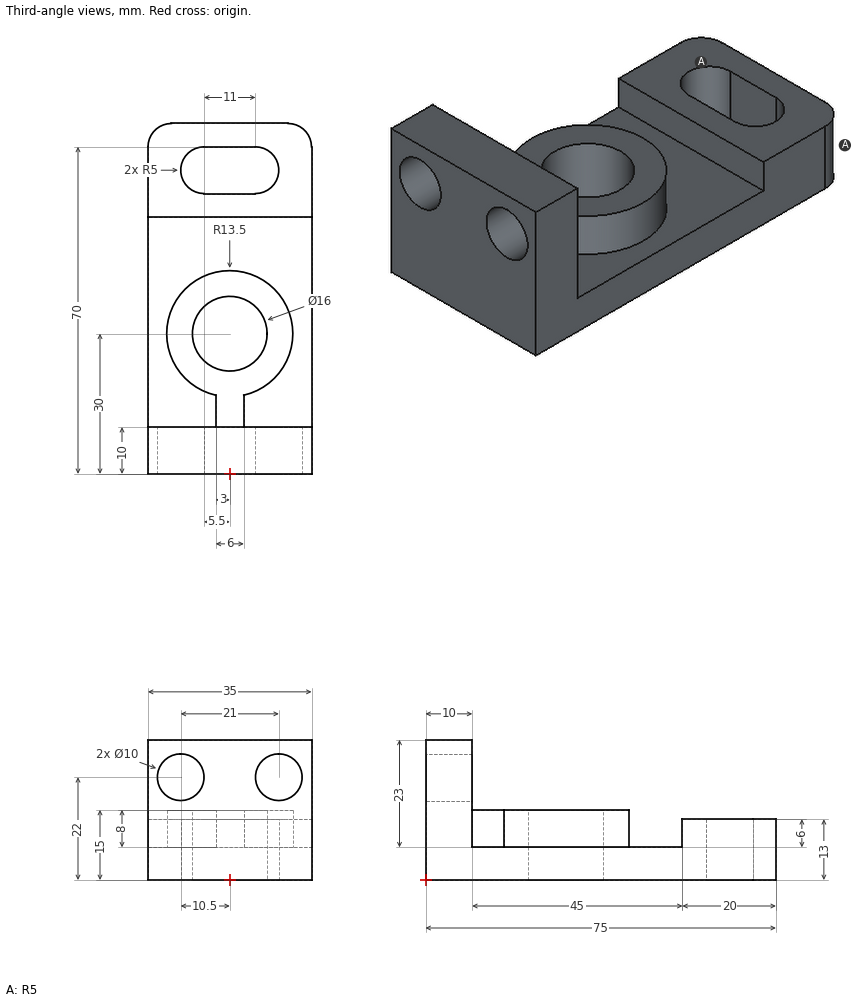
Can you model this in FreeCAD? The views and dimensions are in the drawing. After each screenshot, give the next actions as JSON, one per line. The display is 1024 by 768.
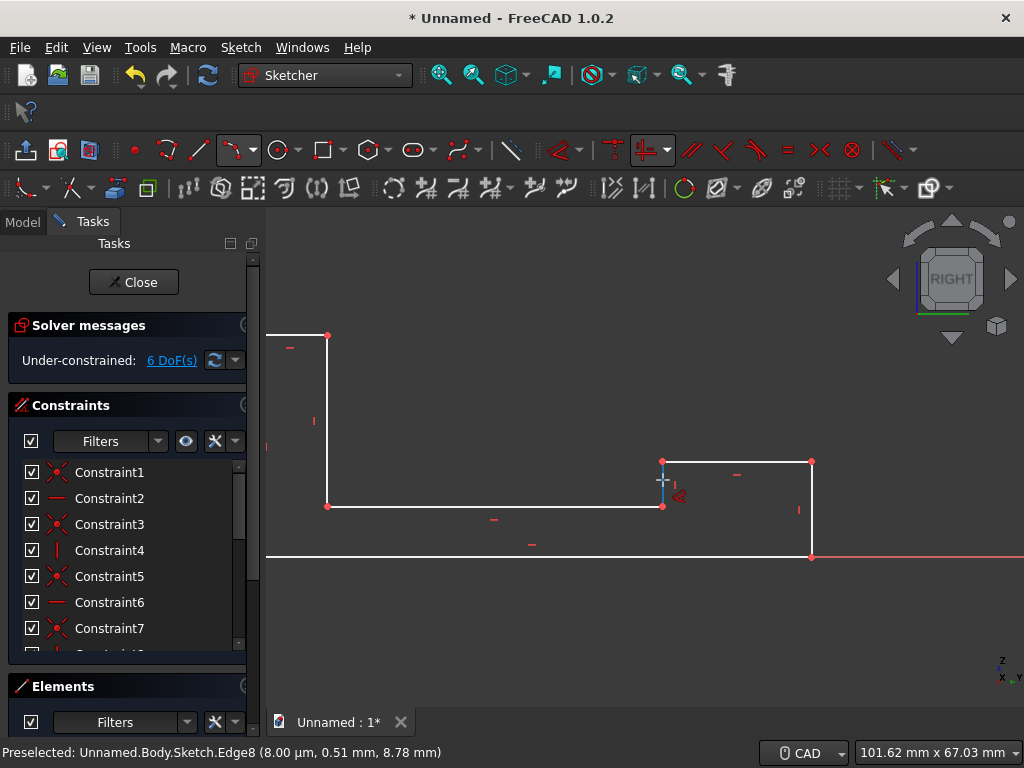
{"action": "left_click", "coordinate": [663, 480]}
{"action": "left_click", "coordinate": [697, 484]}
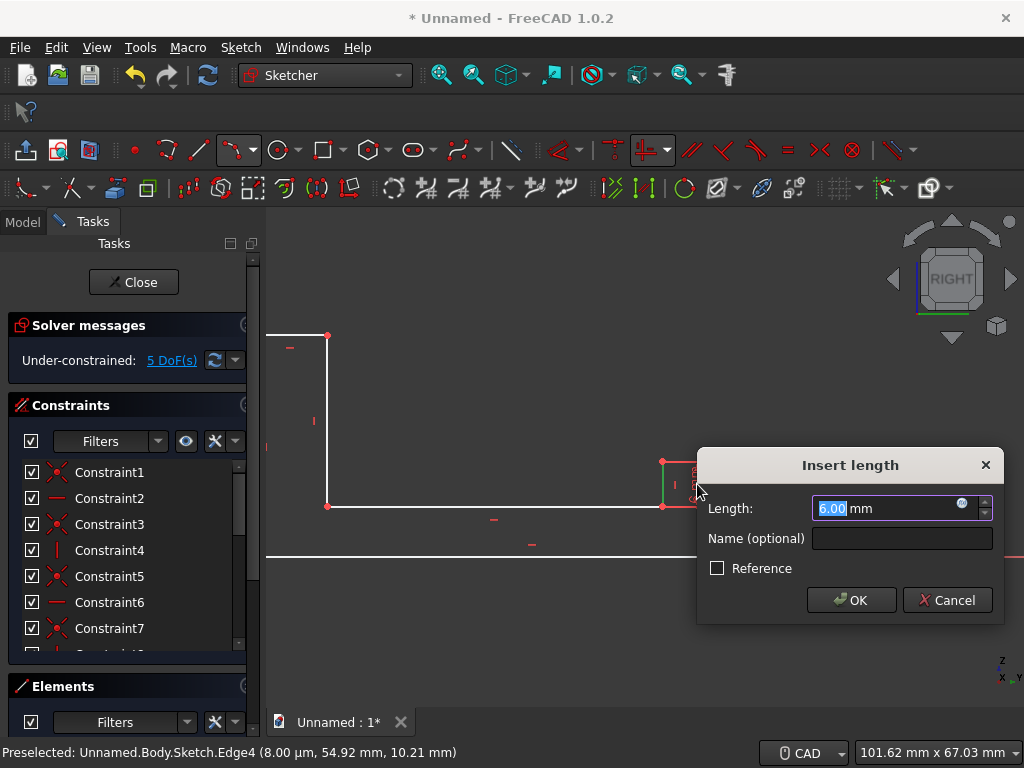
{"action": "type", "text": "6"}
{"action": "key", "text": "Return"}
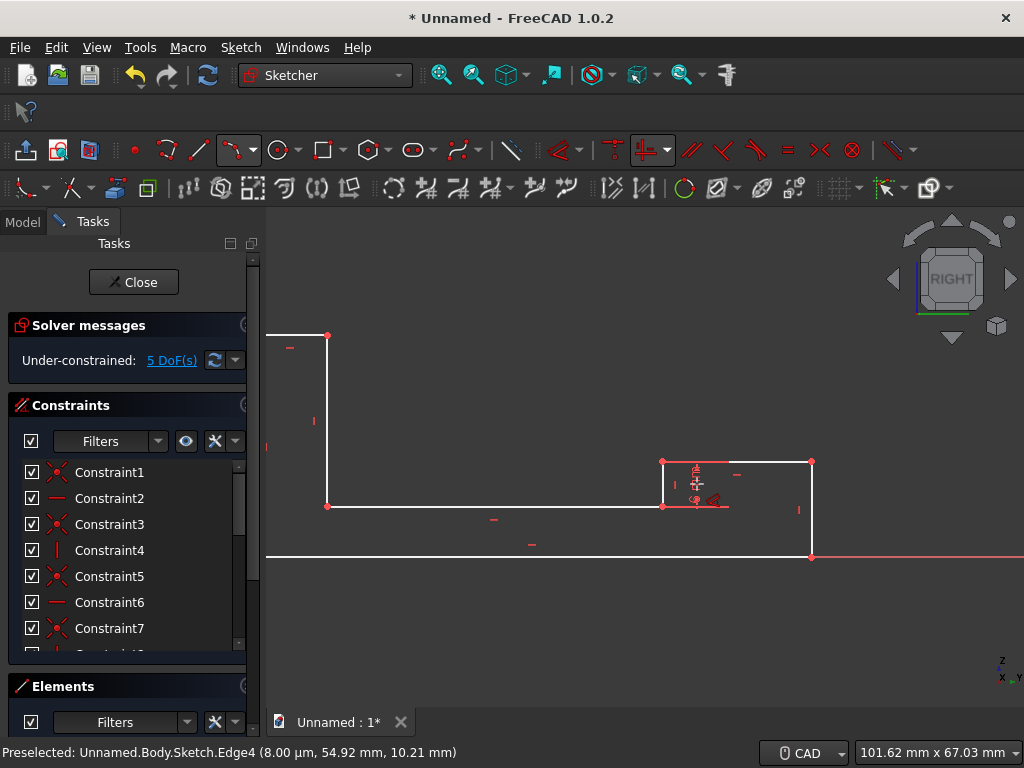
{"action": "left_click", "coordinate": [421, 557]}
{"action": "left_click", "coordinate": [553, 591]}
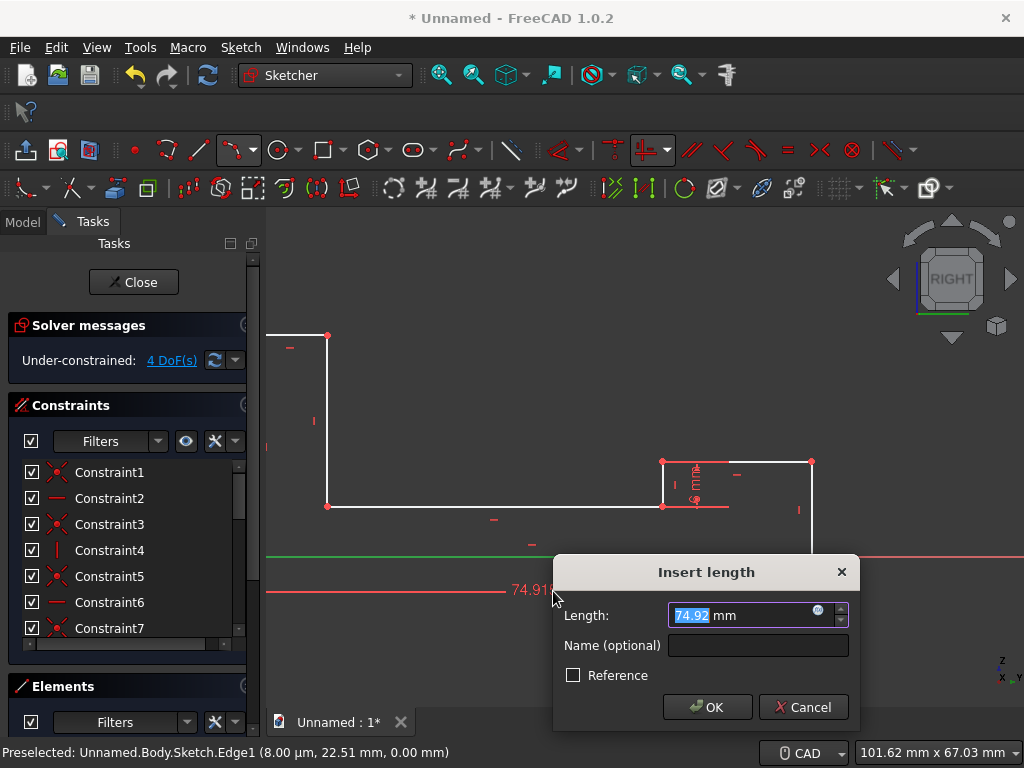
{"action": "type", "text": "75"}
{"action": "key", "text": "Return"}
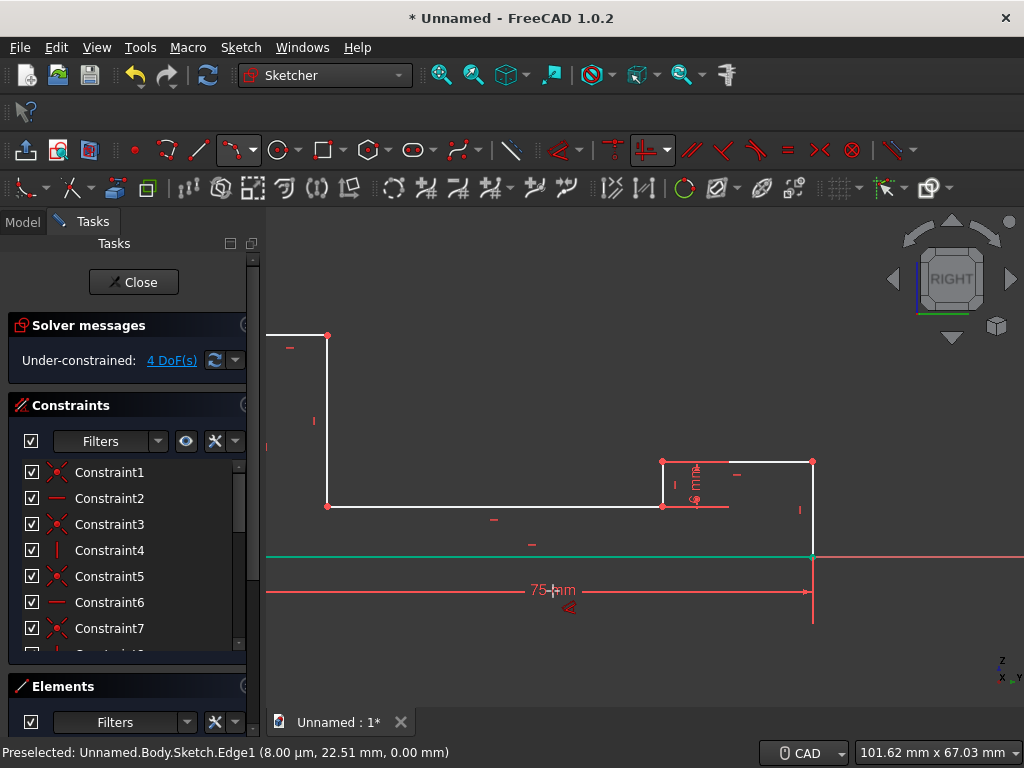
{"action": "left_click", "coordinate": [813, 529]}
{"action": "left_click", "coordinate": [847, 509]}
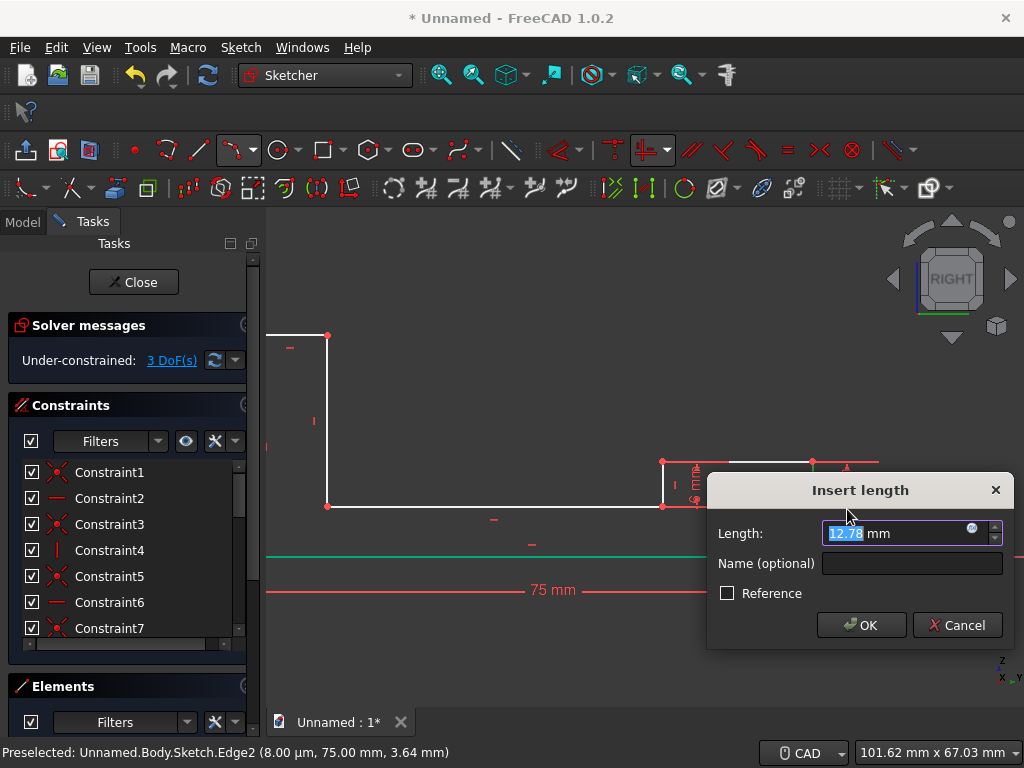
{"action": "type", "text": "13"}
{"action": "key", "text": "Return"}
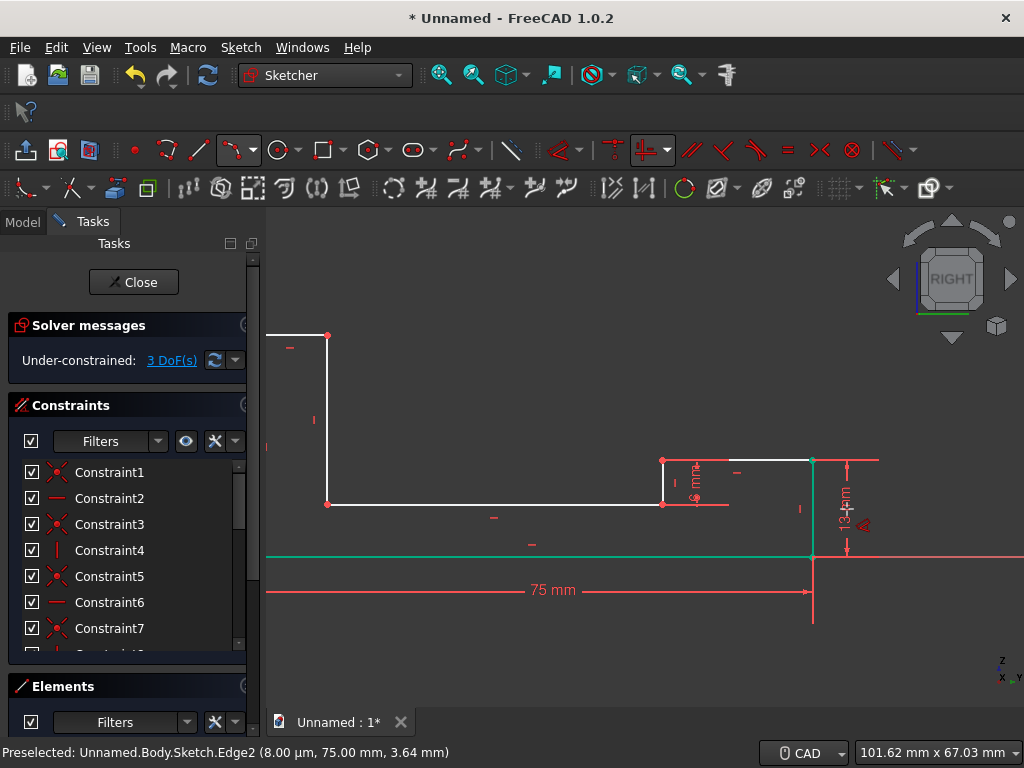
{"action": "left_click", "coordinate": [768, 460]}
{"action": "left_click", "coordinate": [772, 494]}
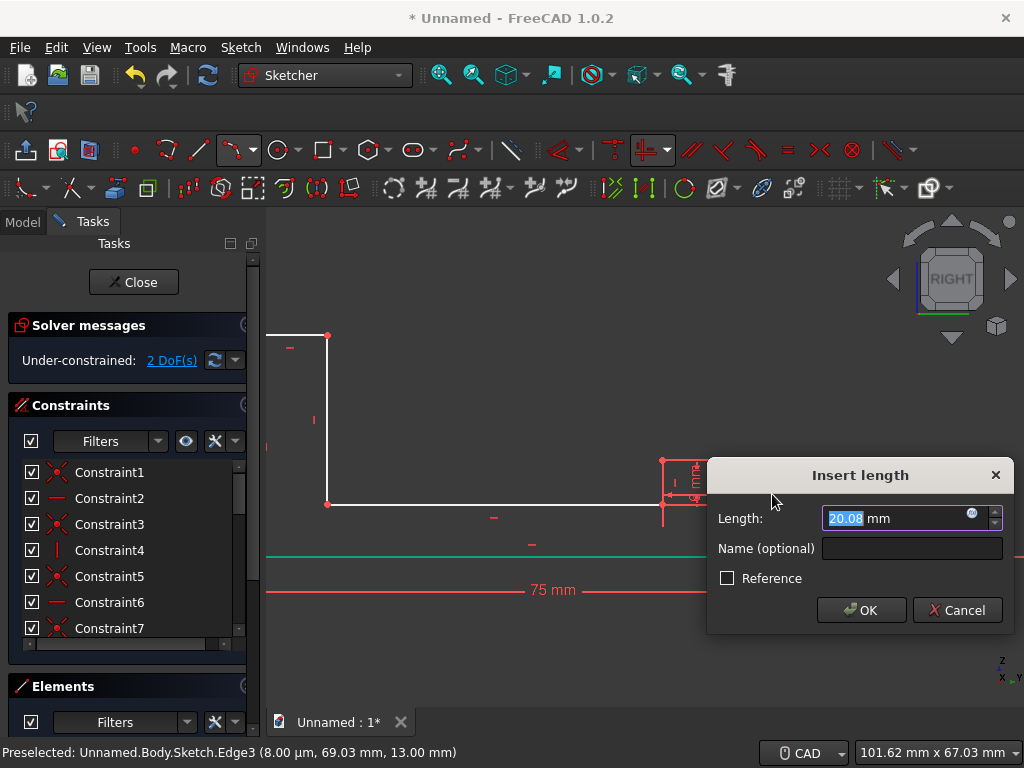
{"action": "type", "text": "20"}
{"action": "key", "text": "Return"}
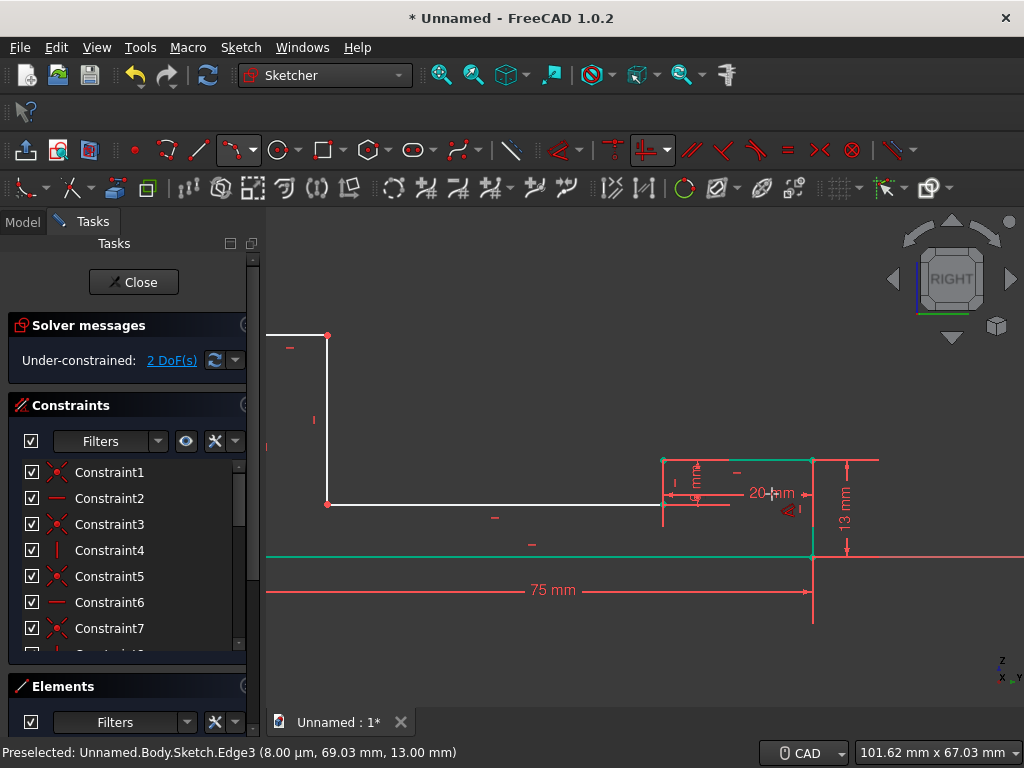
{"action": "left_click", "coordinate": [562, 505]}
{"action": "left_click", "coordinate": [495, 539]}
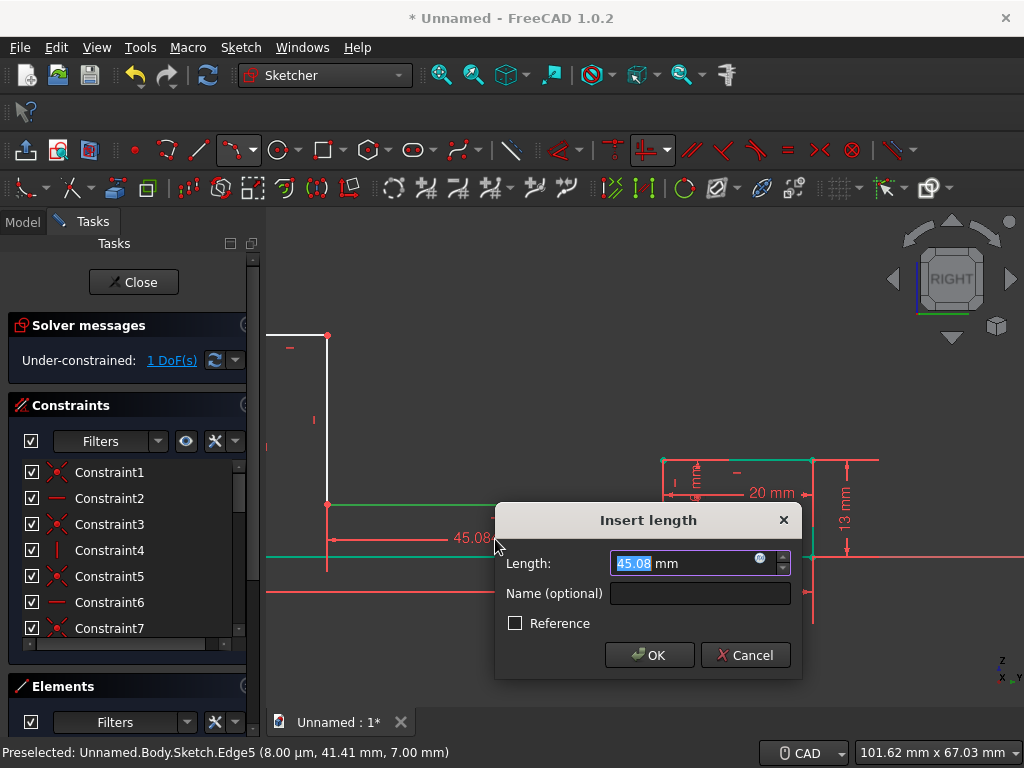
{"action": "type", "text": "45"}
{"action": "key", "text": "Return"}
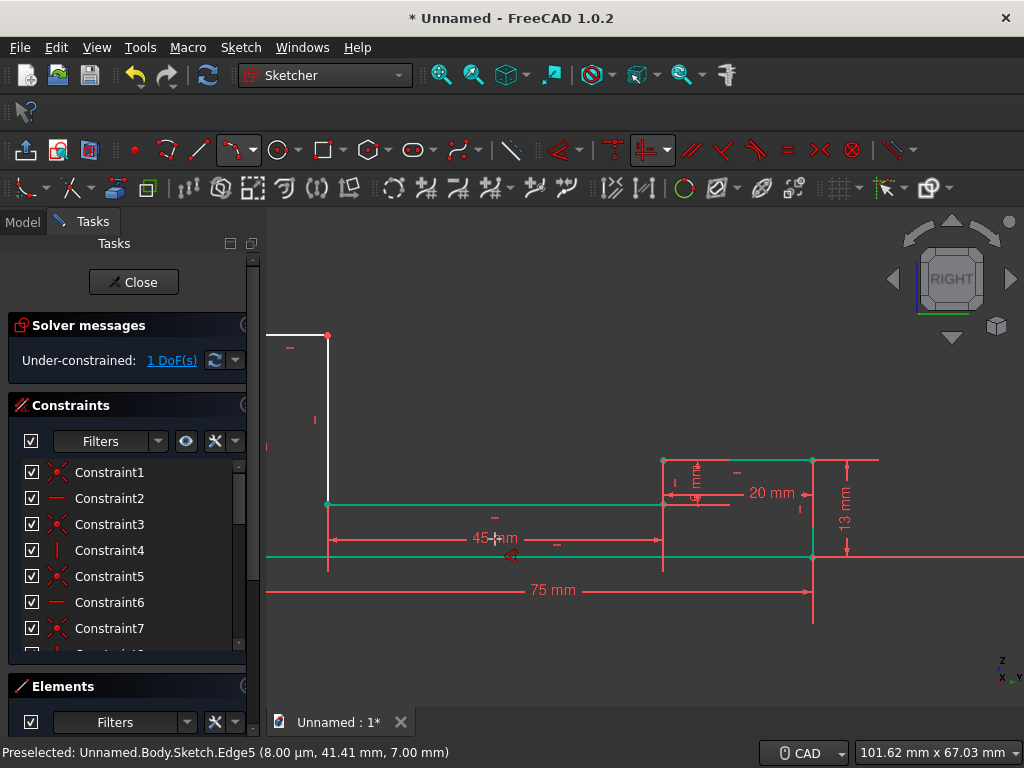
{"action": "left_click", "coordinate": [328, 454]}
{"action": "left_click", "coordinate": [362, 420]}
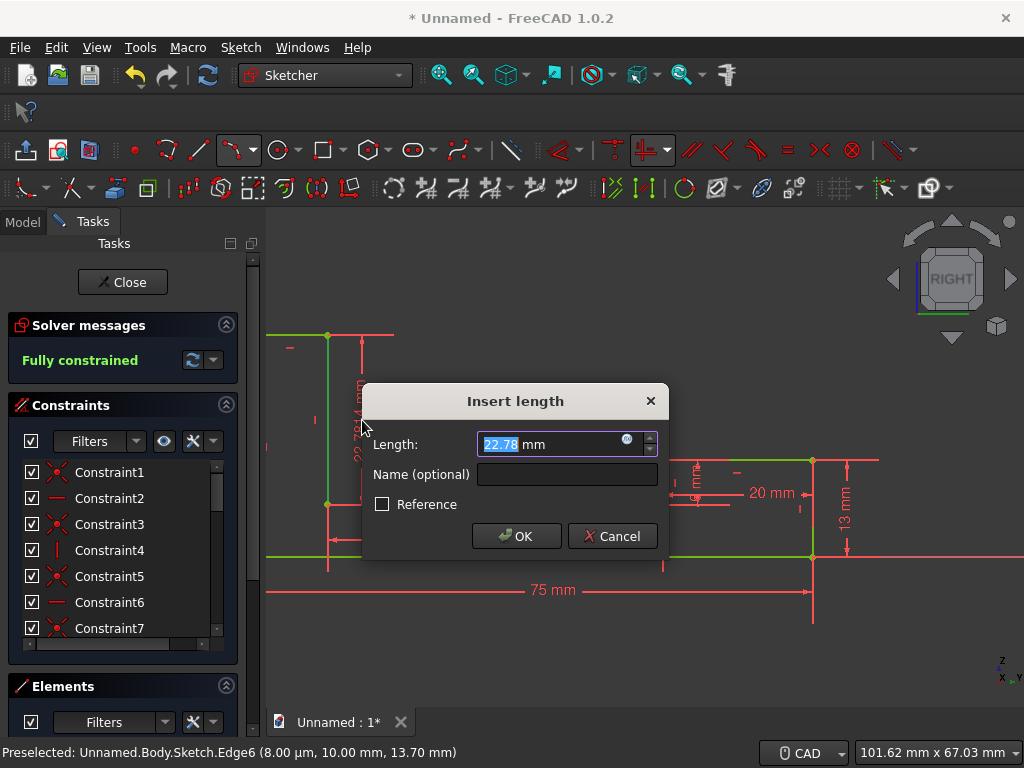
{"action": "type", "text": "23"}
{"action": "key", "text": "Return"}
{"action": "key", "text": "Escape"}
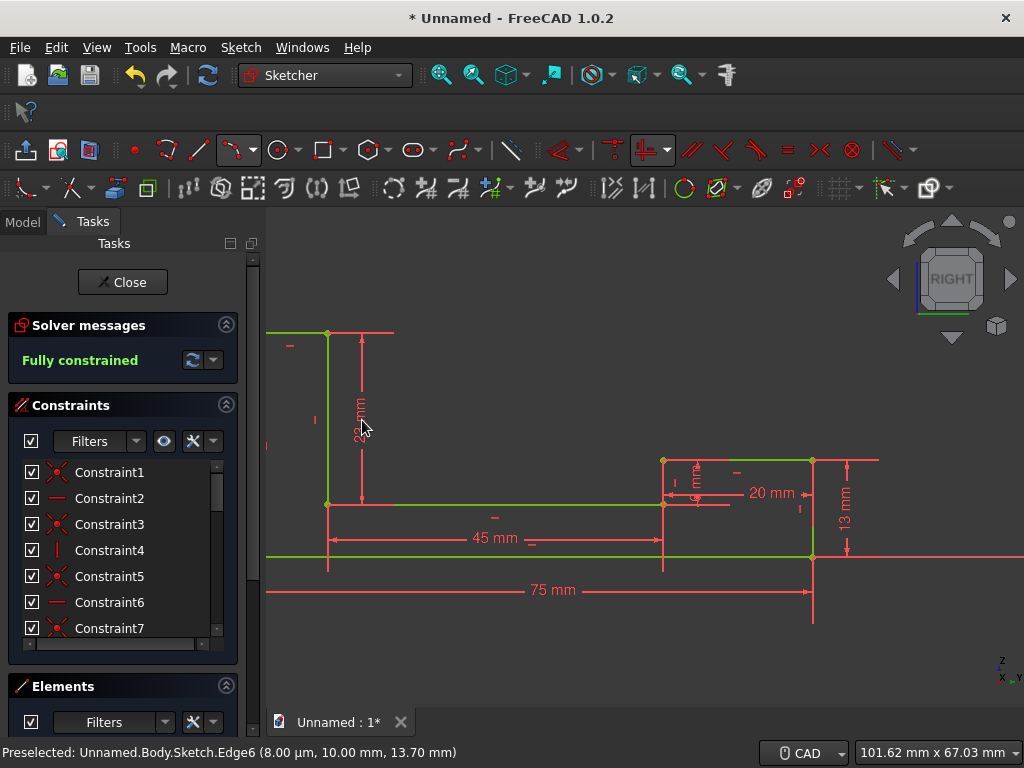
{"action": "left_click", "coordinate": [123, 282]}